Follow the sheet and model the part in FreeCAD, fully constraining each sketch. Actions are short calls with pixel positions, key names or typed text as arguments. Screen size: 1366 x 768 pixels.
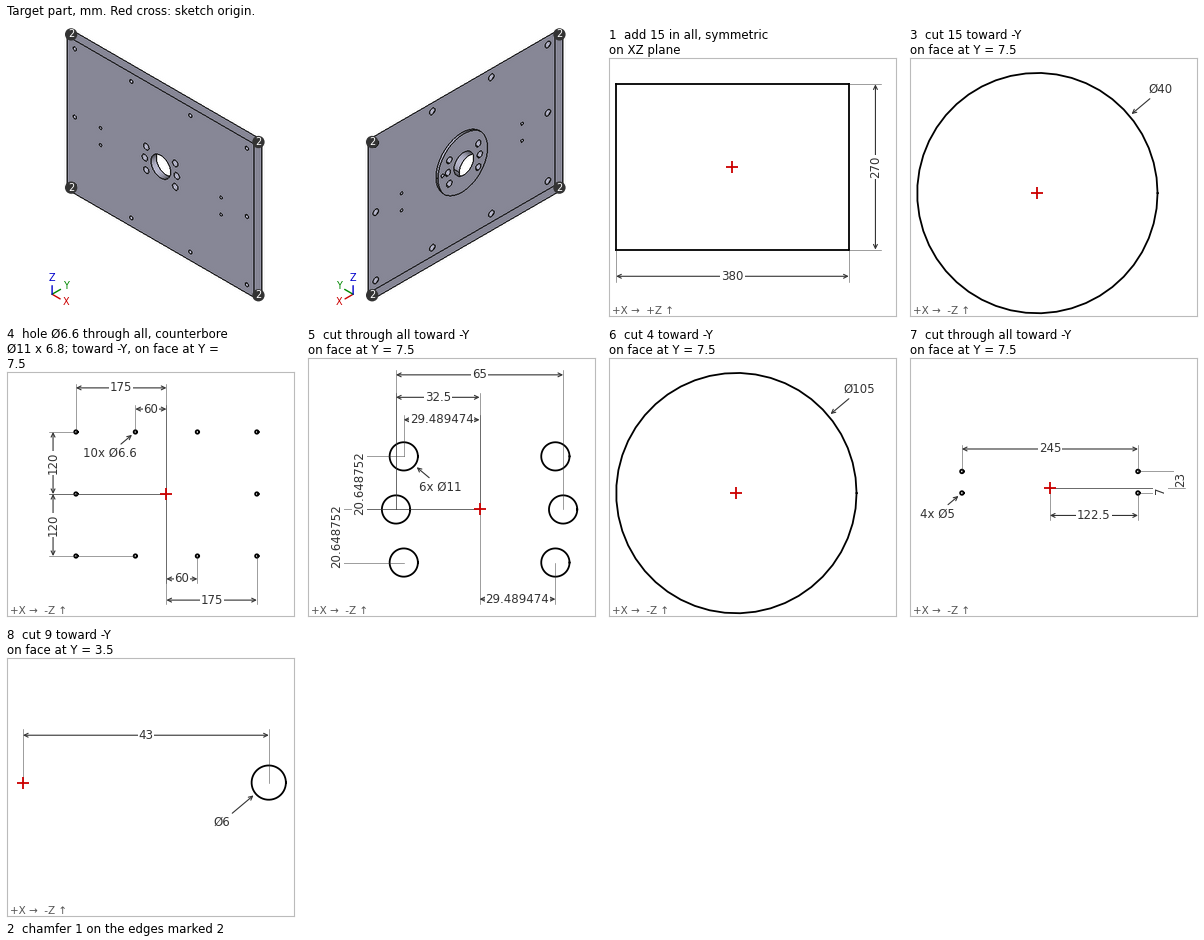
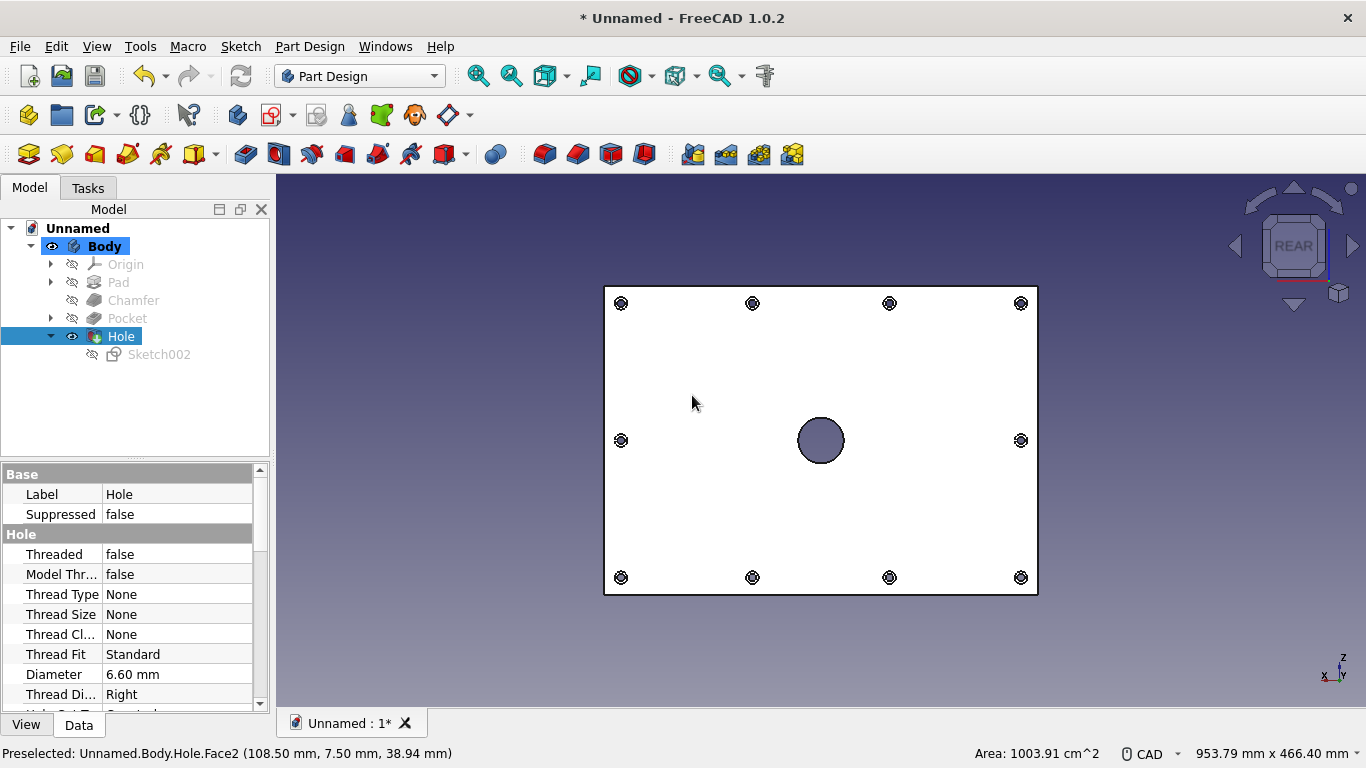
click(270, 116)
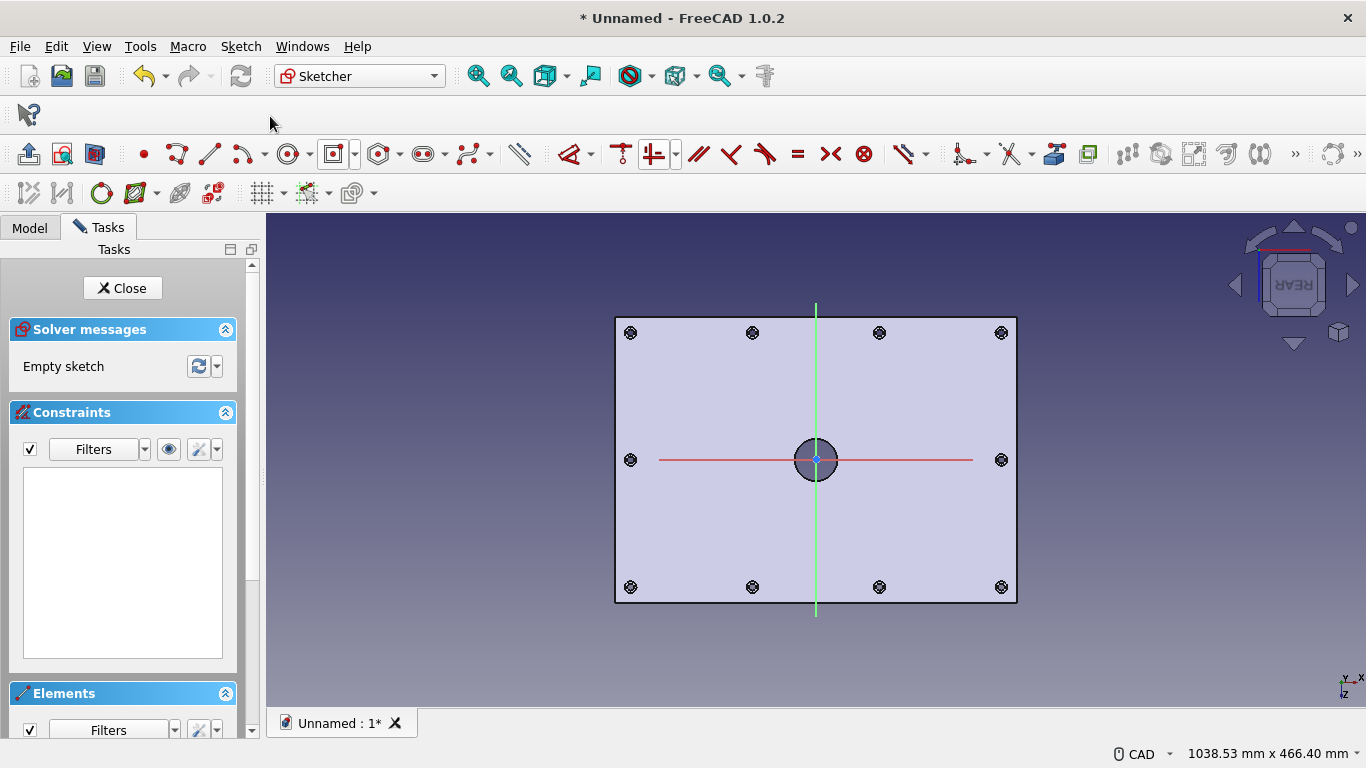
scroll(830, 460, up, 9)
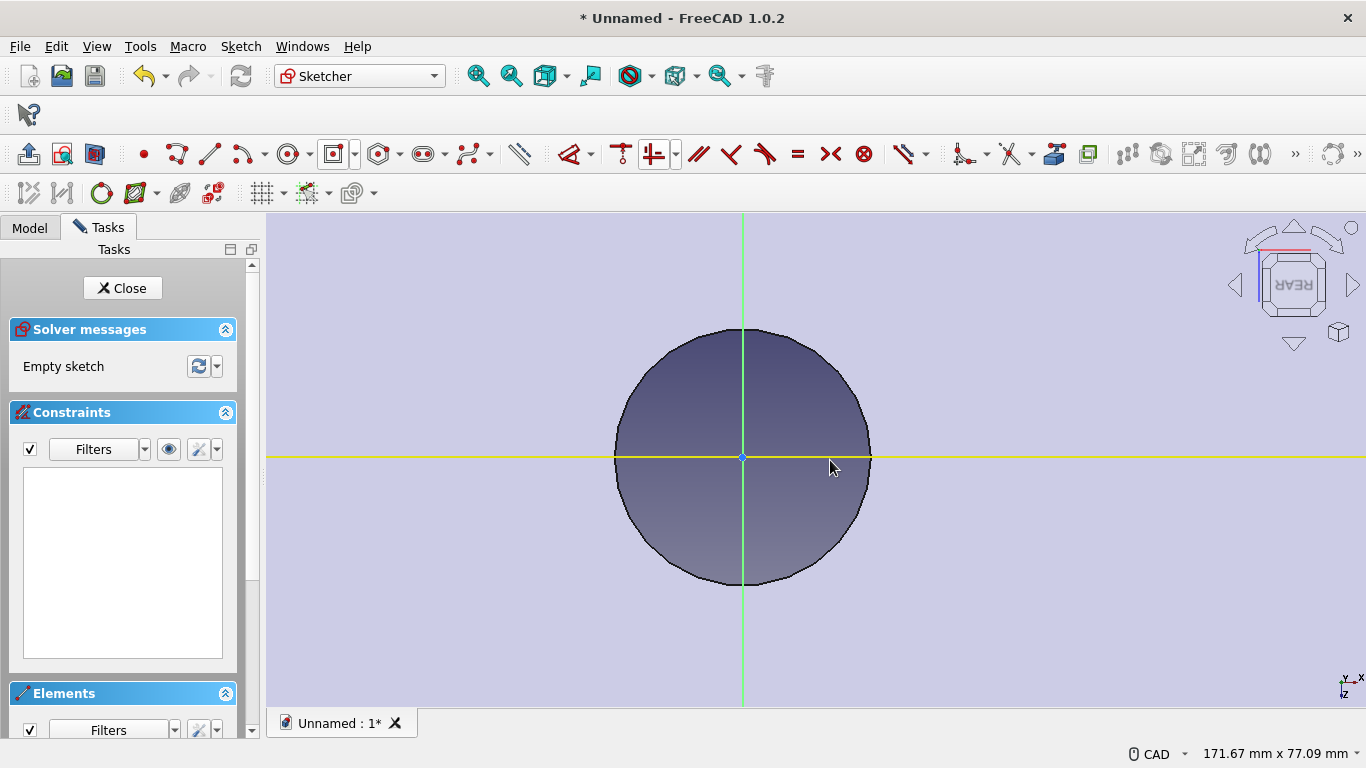
click(288, 154)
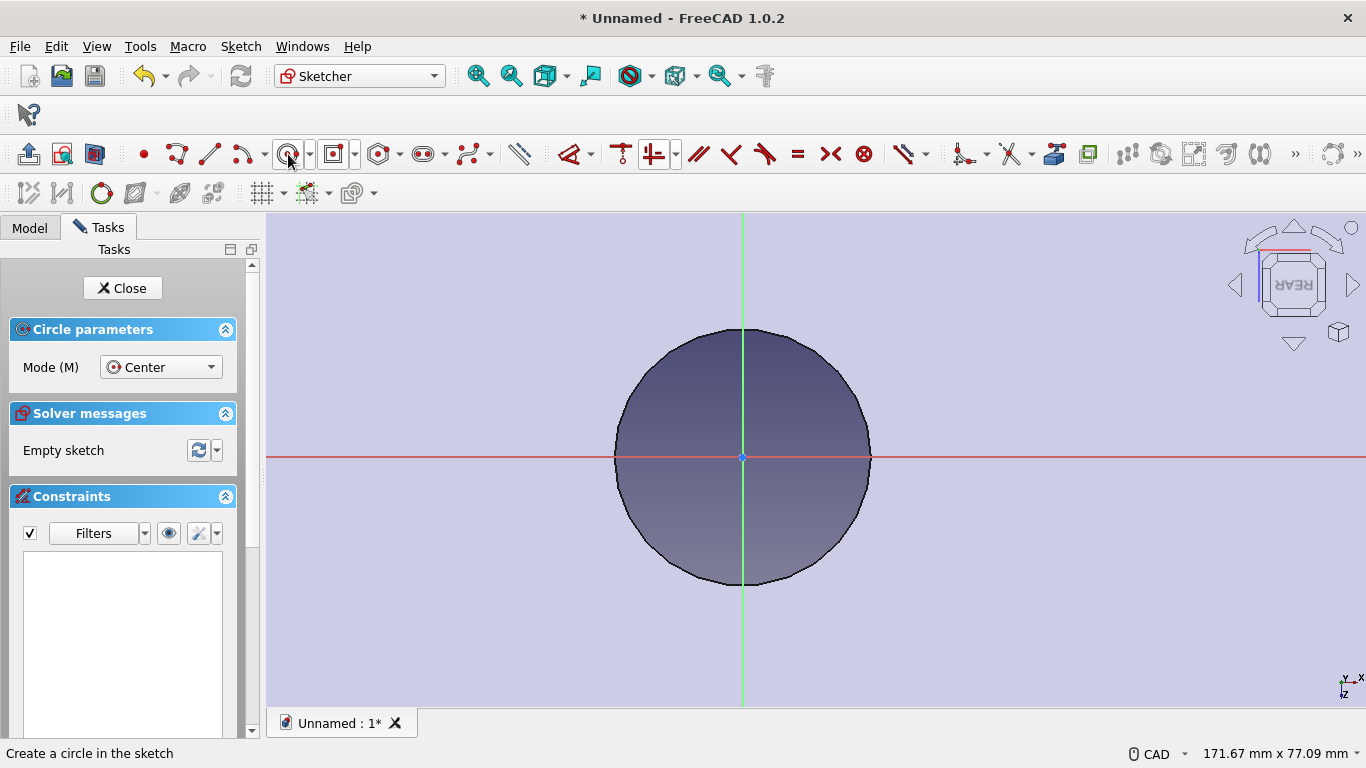
click(554, 325)
click(579, 300)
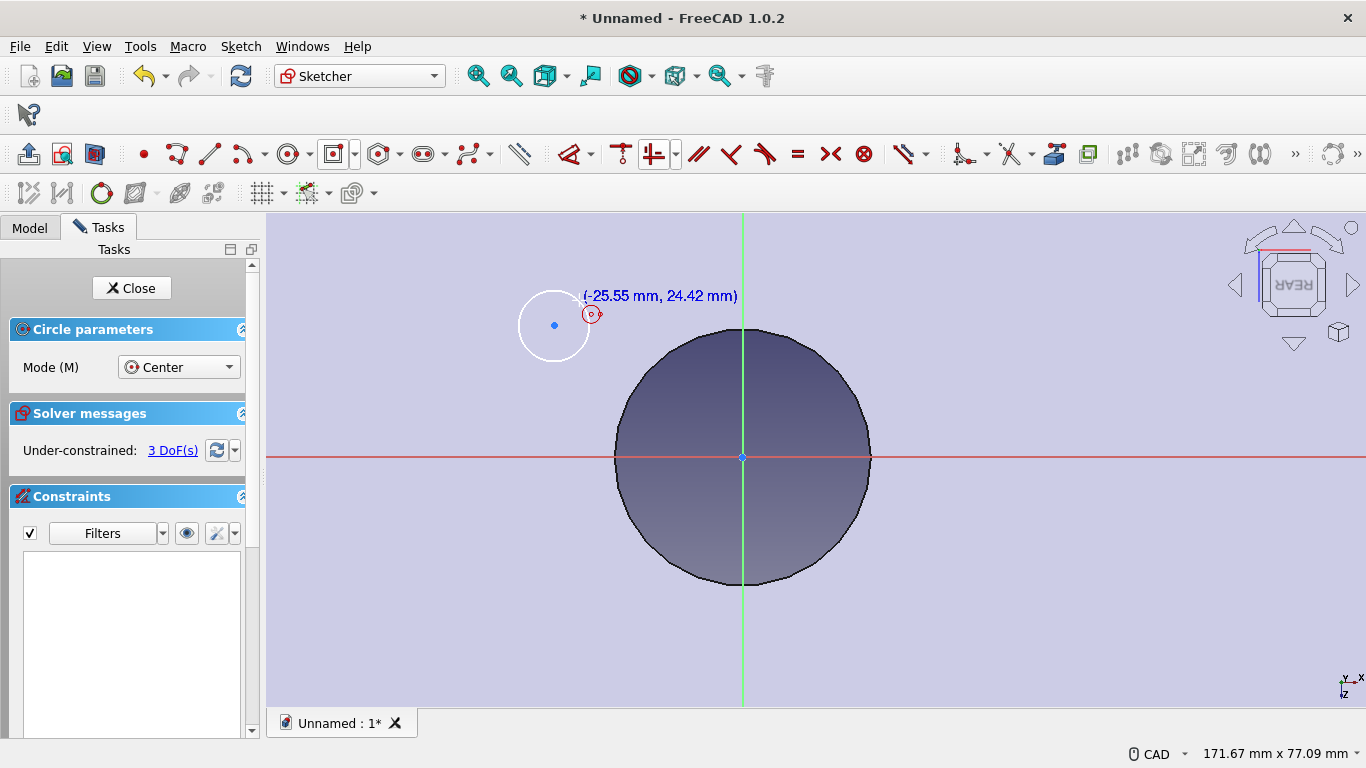
click(554, 590)
click(579, 565)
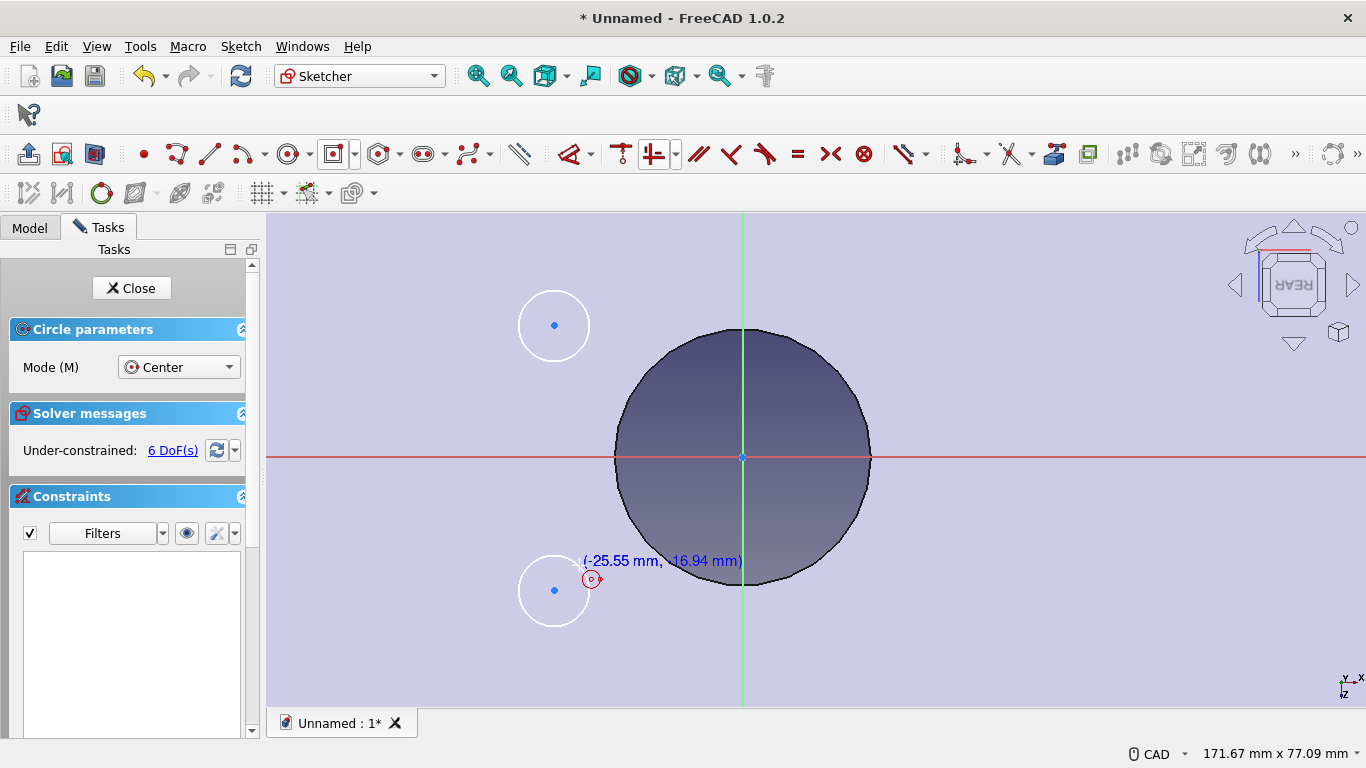
click(534, 457)
click(559, 433)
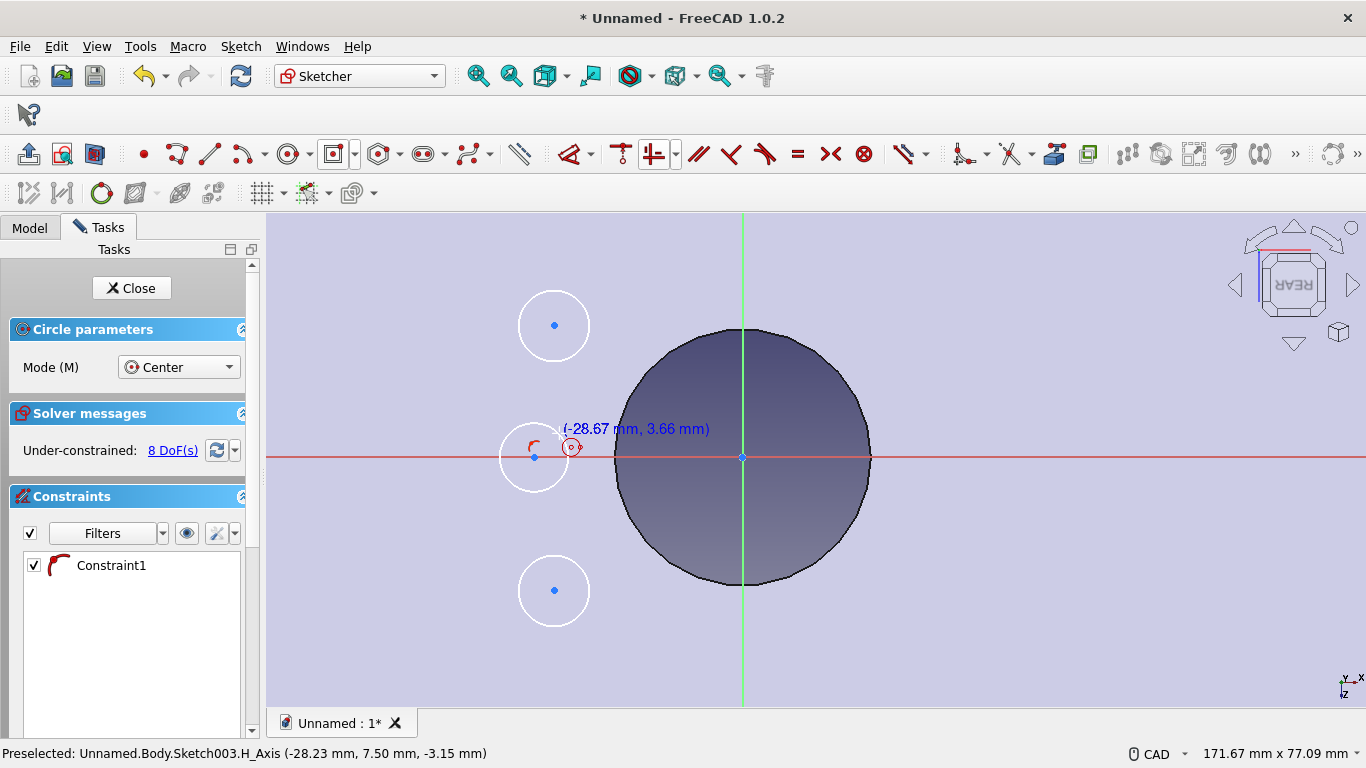
click(932, 590)
click(957, 565)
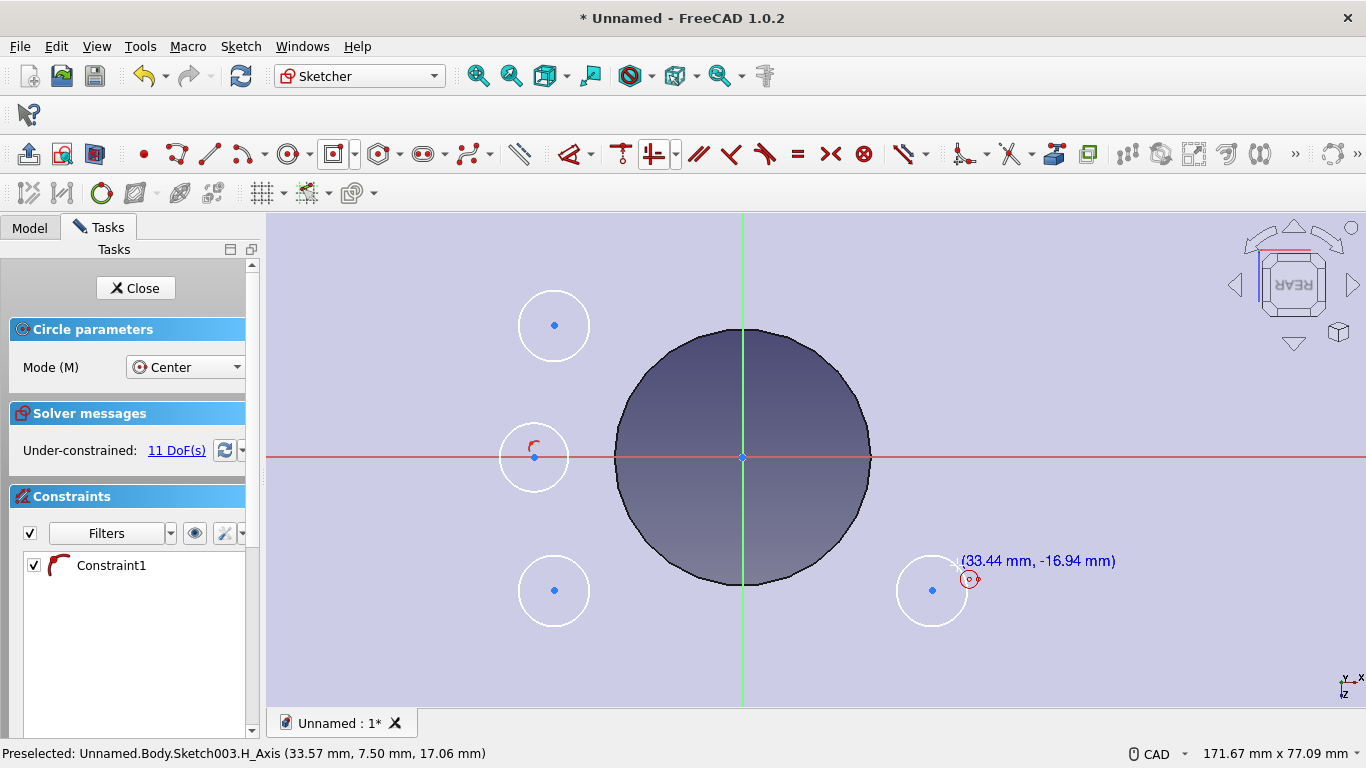
click(951, 457)
click(976, 433)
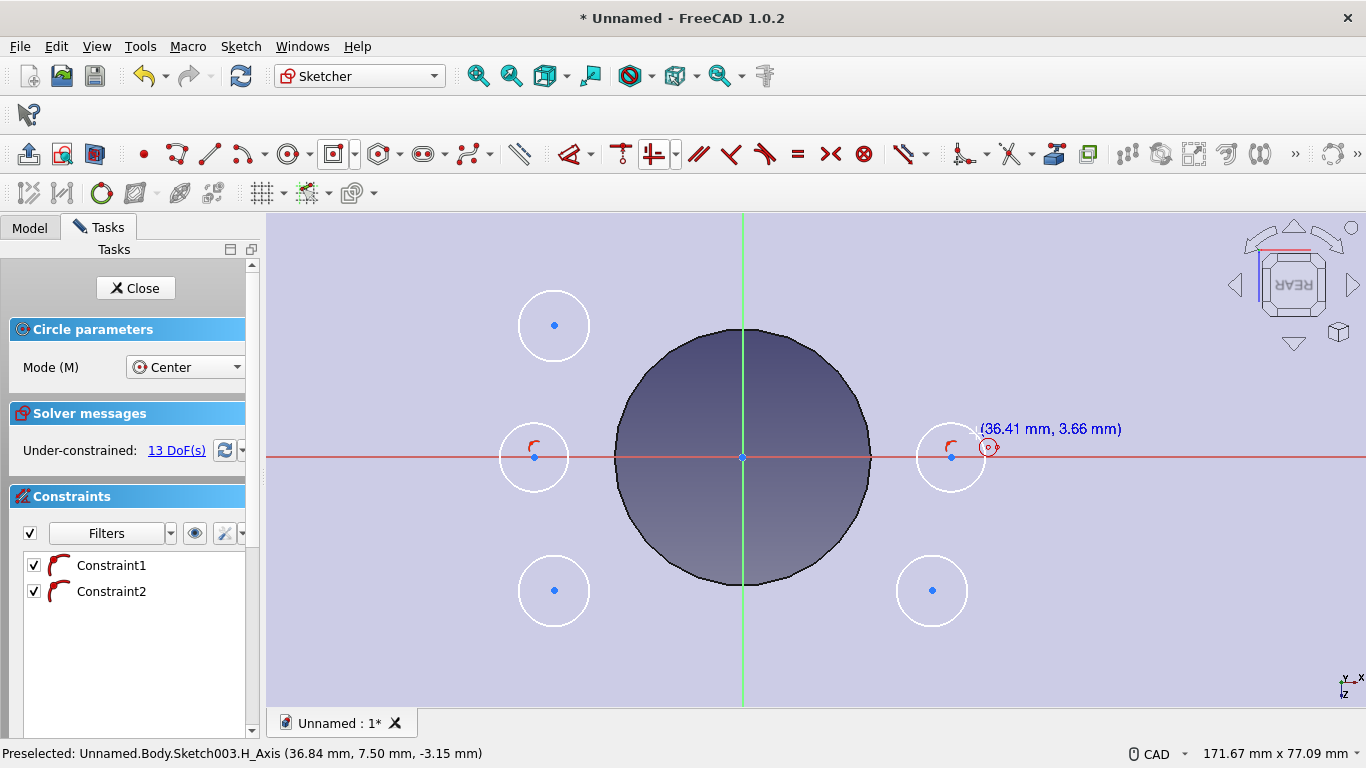
click(932, 325)
click(957, 300)
key(Escape)